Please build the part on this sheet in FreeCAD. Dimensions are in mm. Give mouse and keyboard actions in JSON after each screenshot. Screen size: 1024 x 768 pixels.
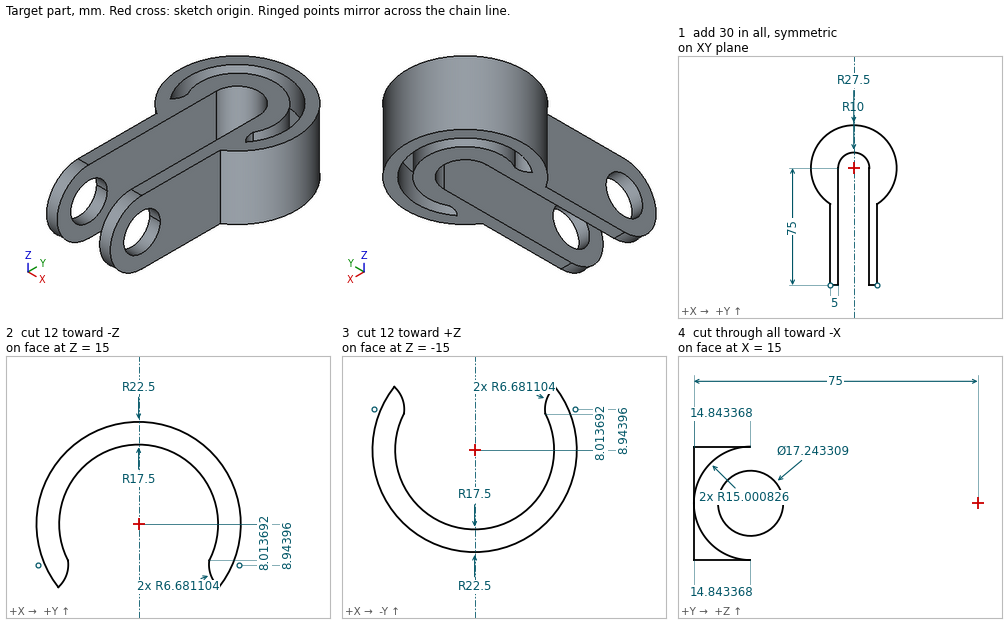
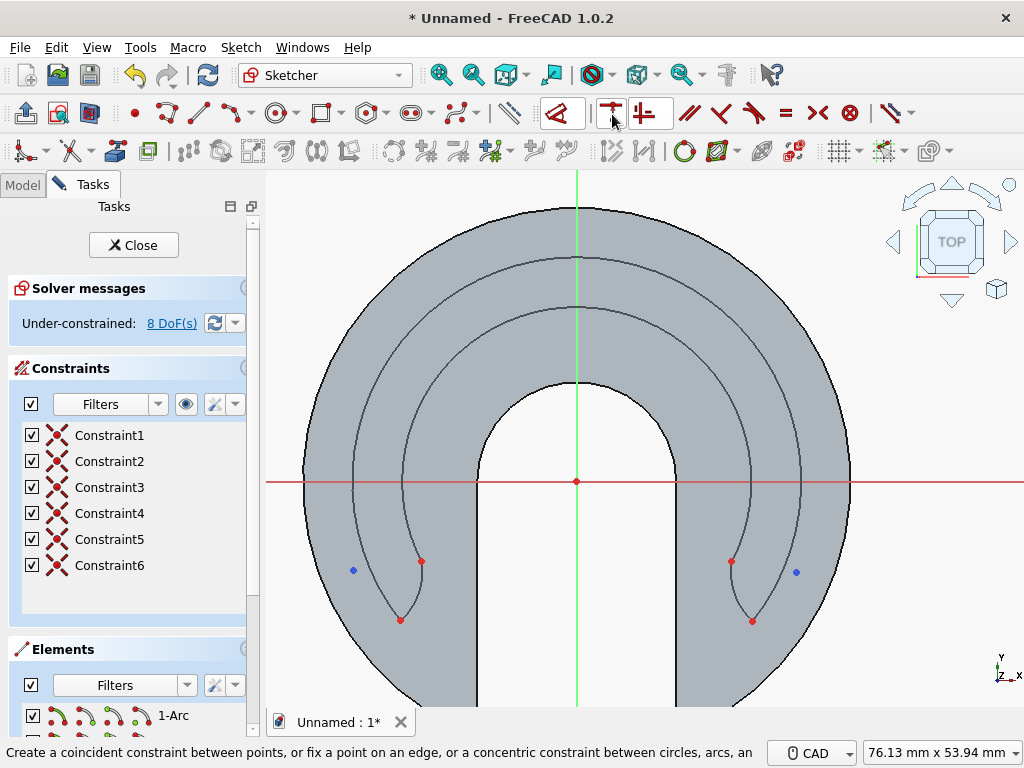
{"action": "left_click", "coordinate": [732, 582]}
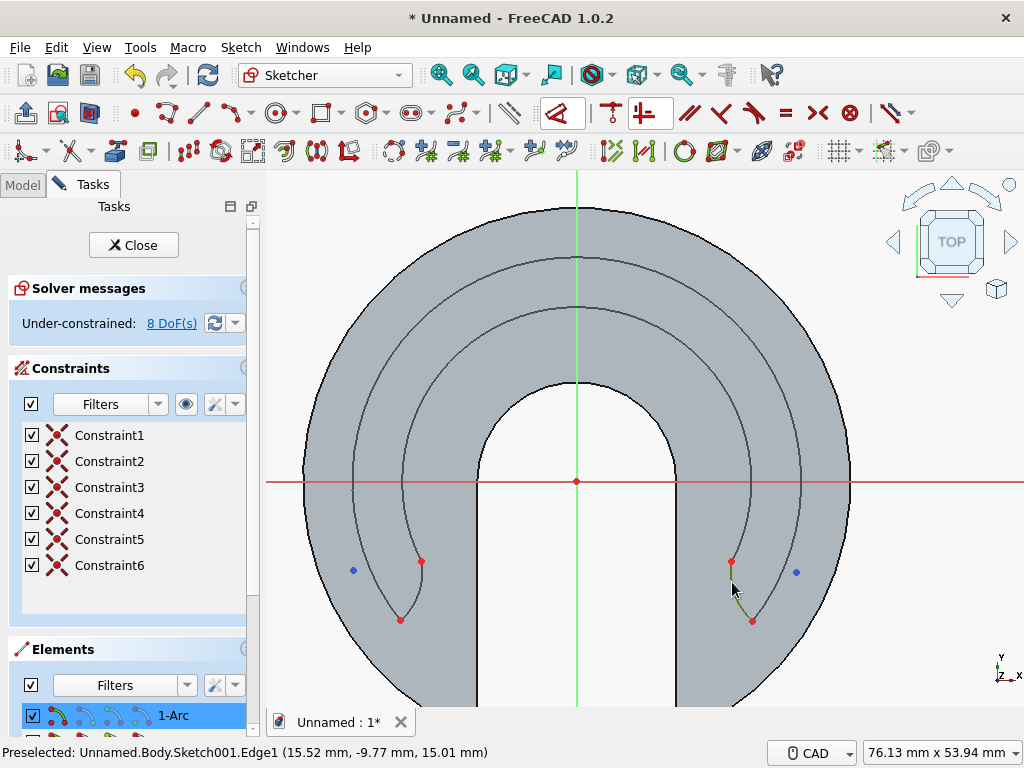
{"action": "left_click", "coordinate": [413, 606]}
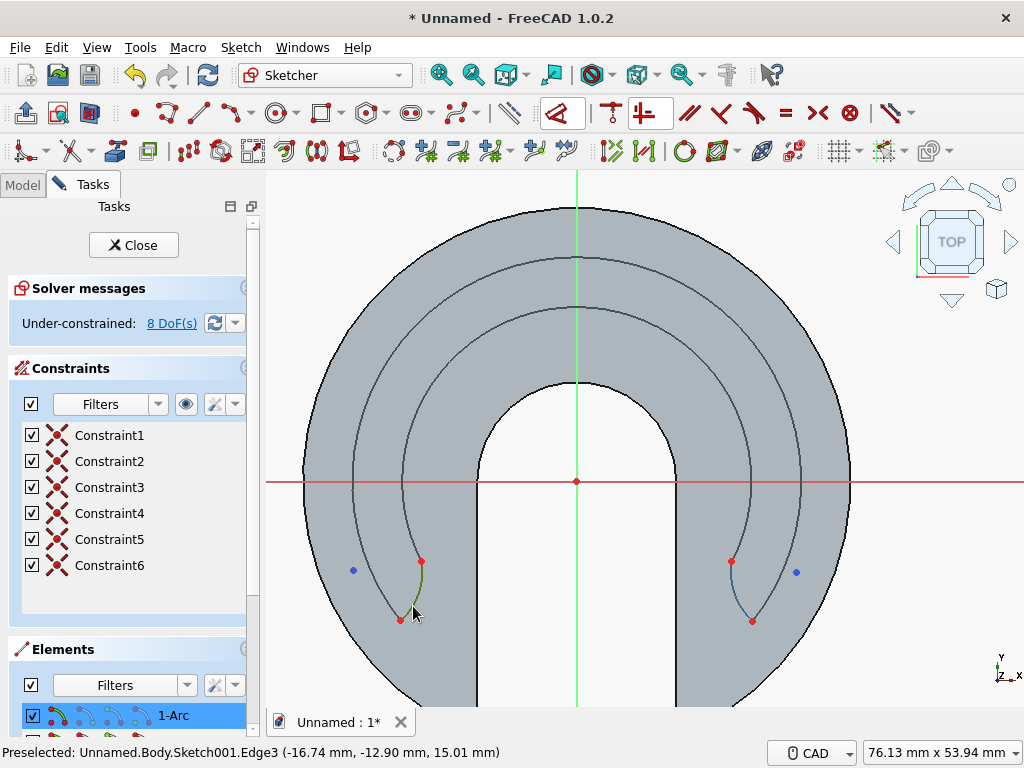
{"action": "left_click", "coordinate": [786, 114]}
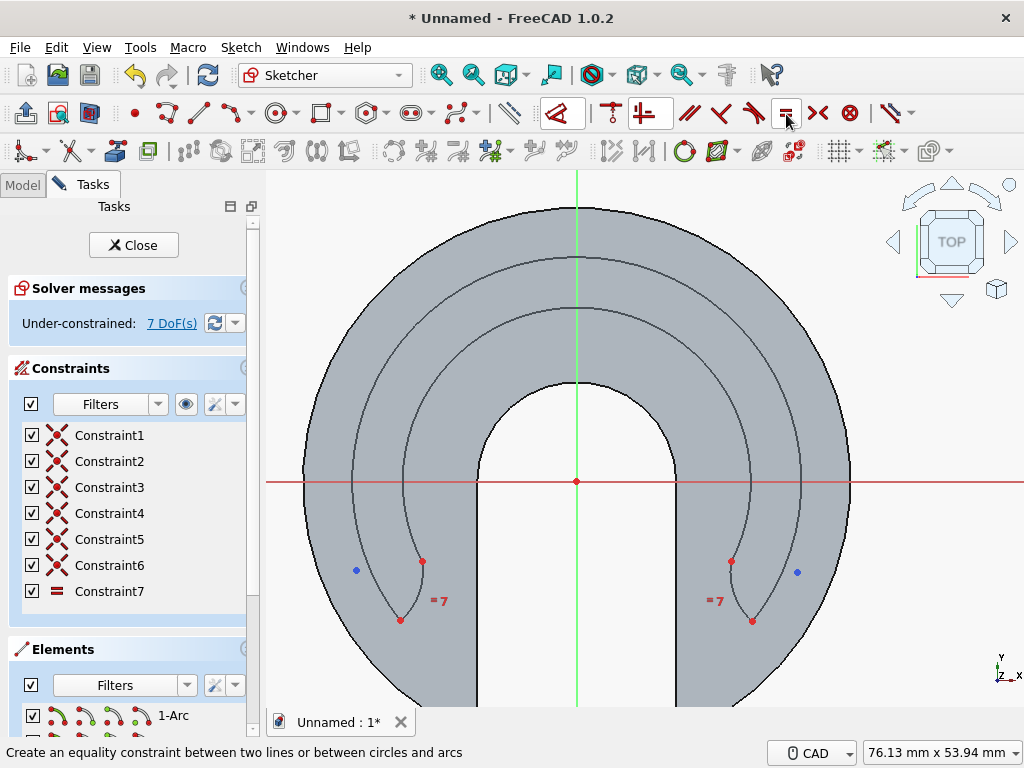
{"action": "left_click", "coordinate": [797, 572]}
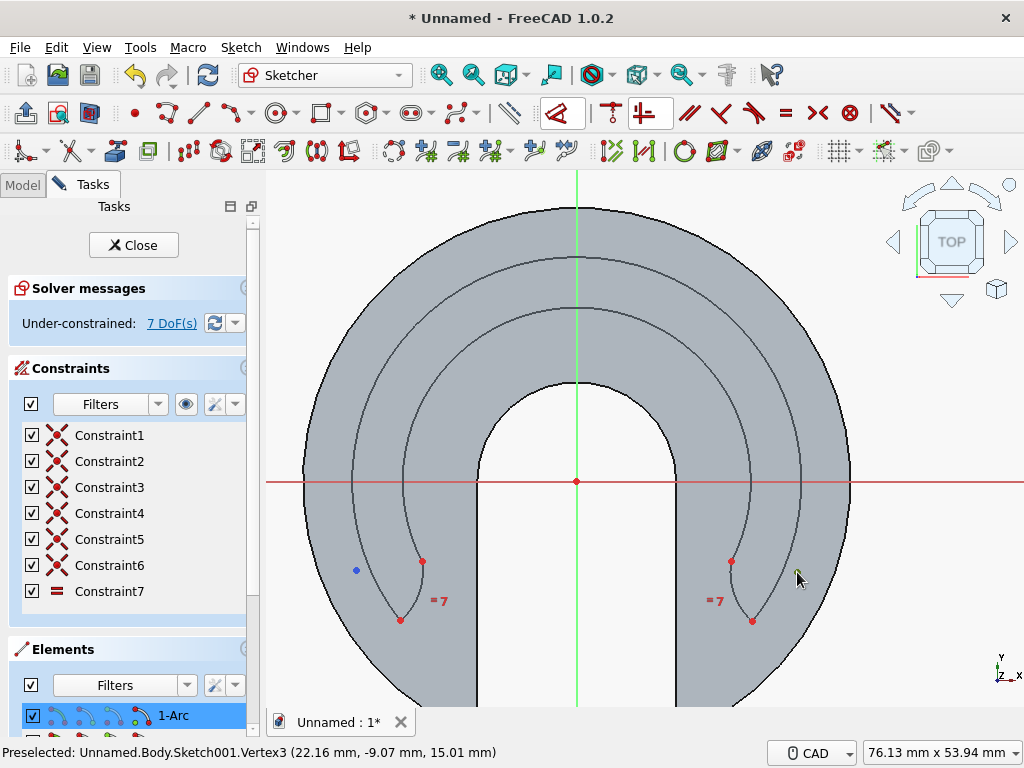
{"action": "left_click", "coordinate": [356, 571]}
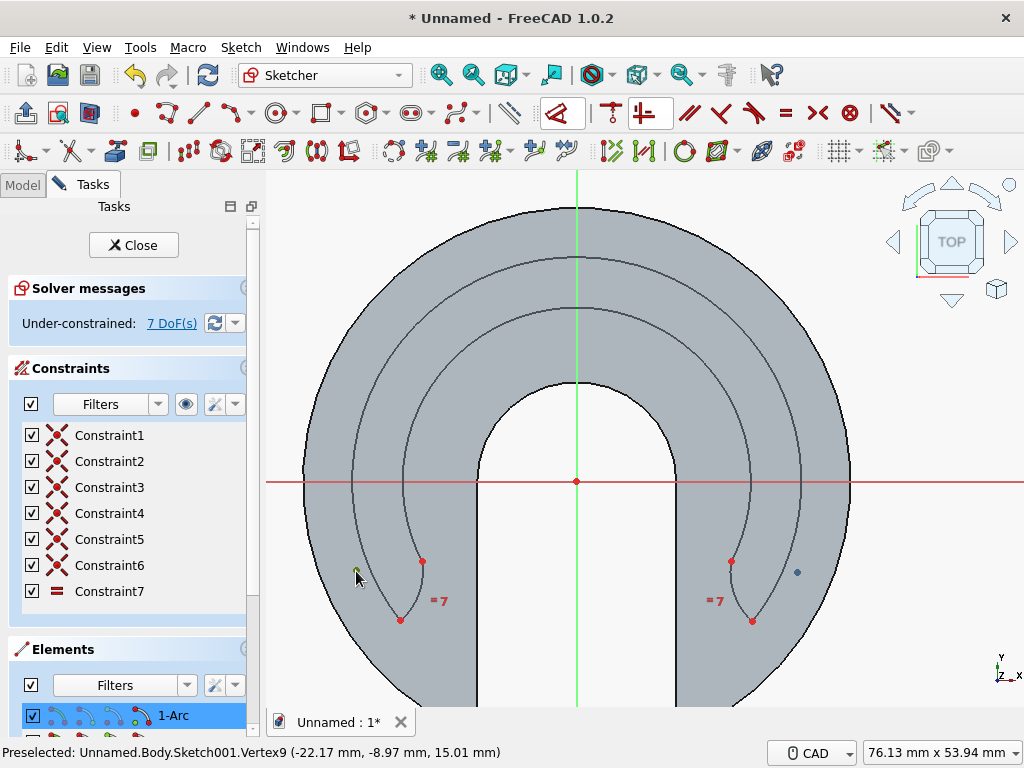
{"action": "left_click", "coordinate": [577, 645]}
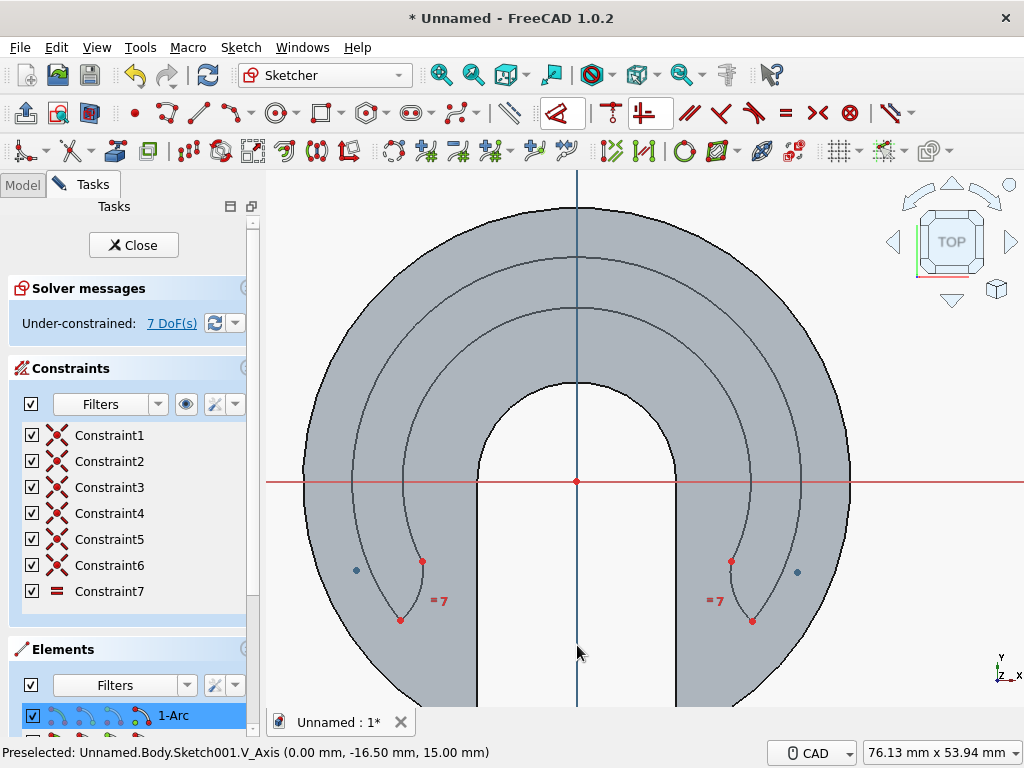
{"action": "key", "text": "s"}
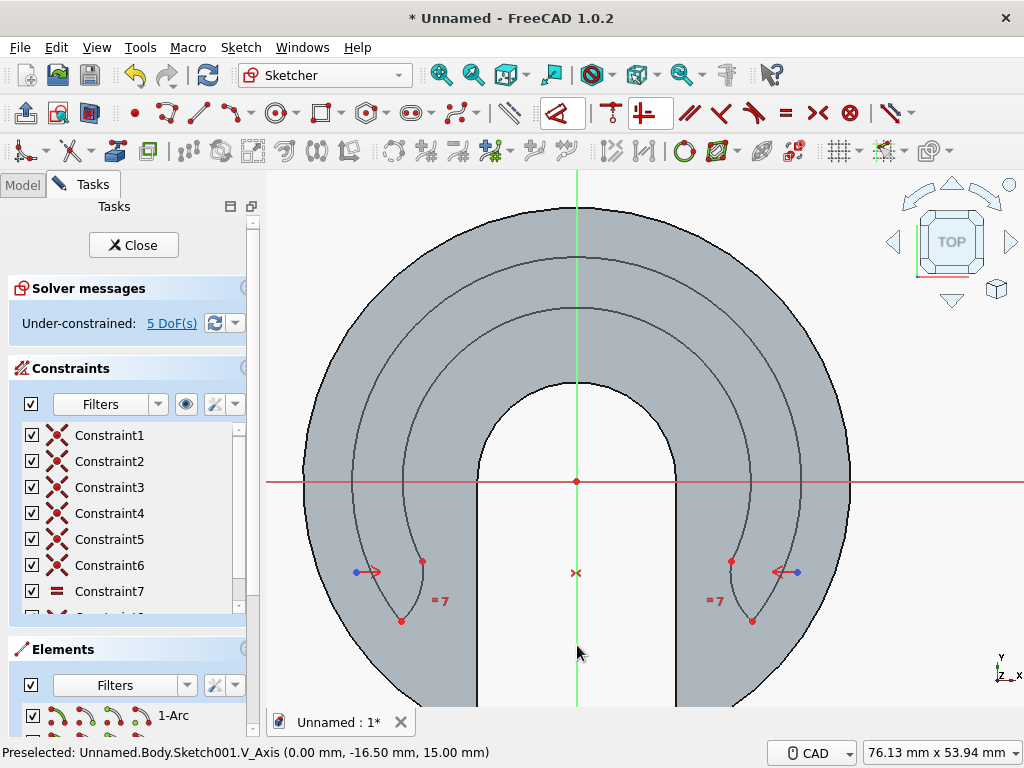
{"action": "left_click", "coordinate": [731, 582]}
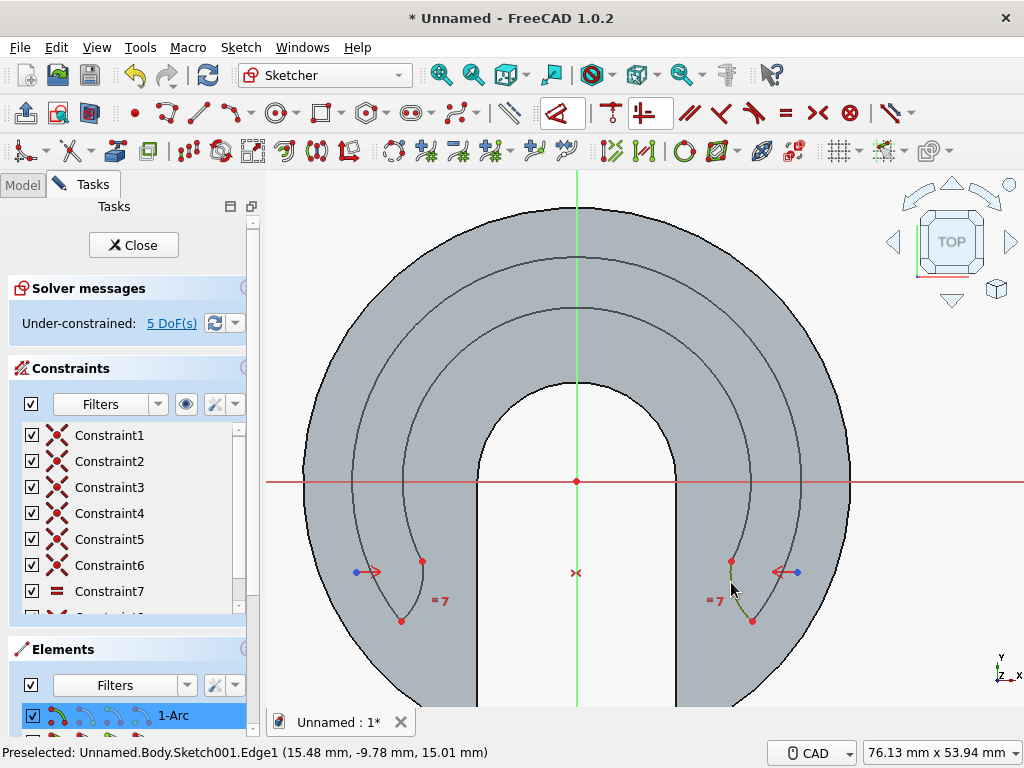
{"action": "left_click", "coordinate": [580, 114]}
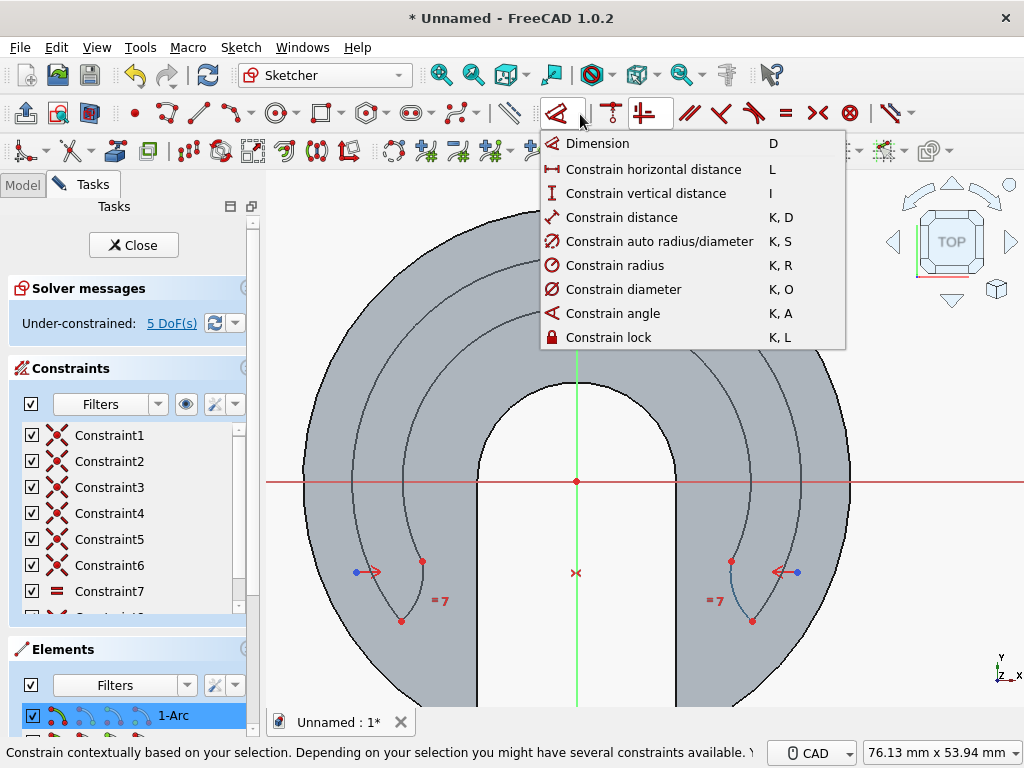
{"action": "left_click", "coordinate": [693, 265]}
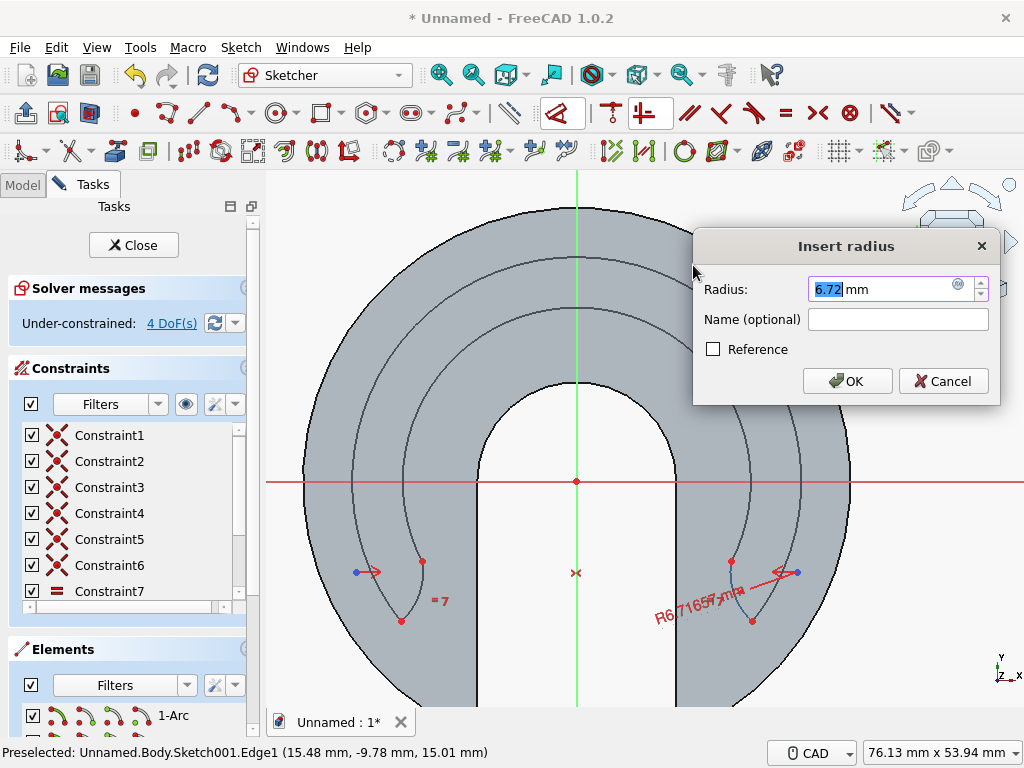
{"action": "type", "text": "6.681104"}
{"action": "key", "text": "Return"}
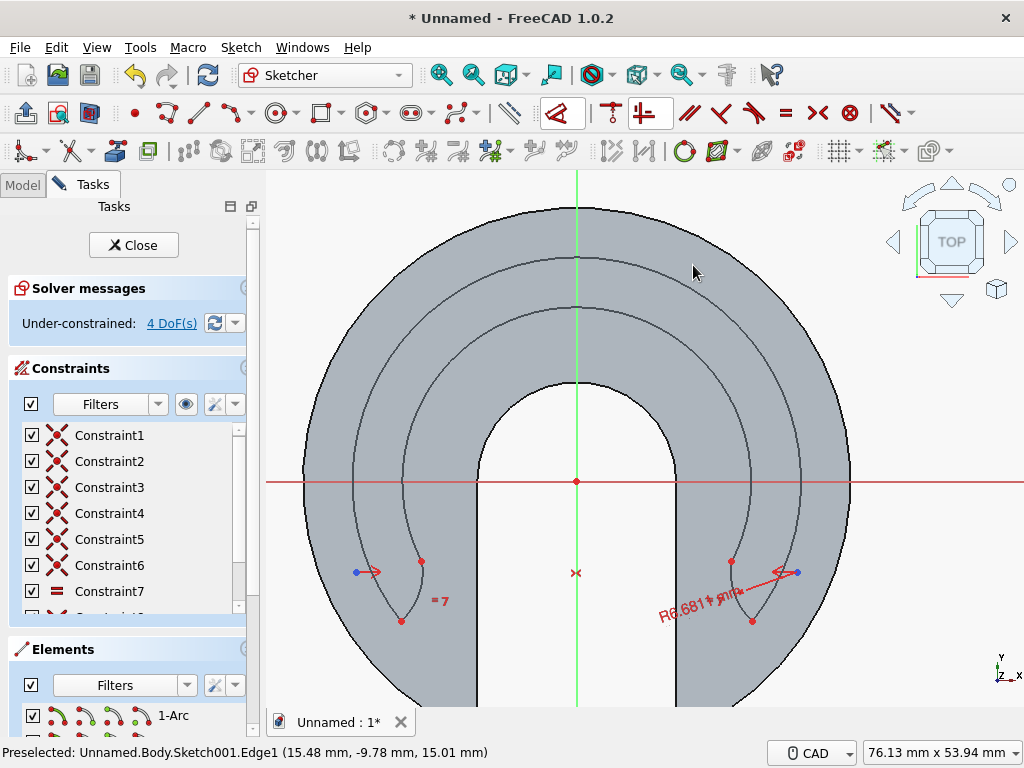
{"action": "left_click", "coordinate": [752, 342]}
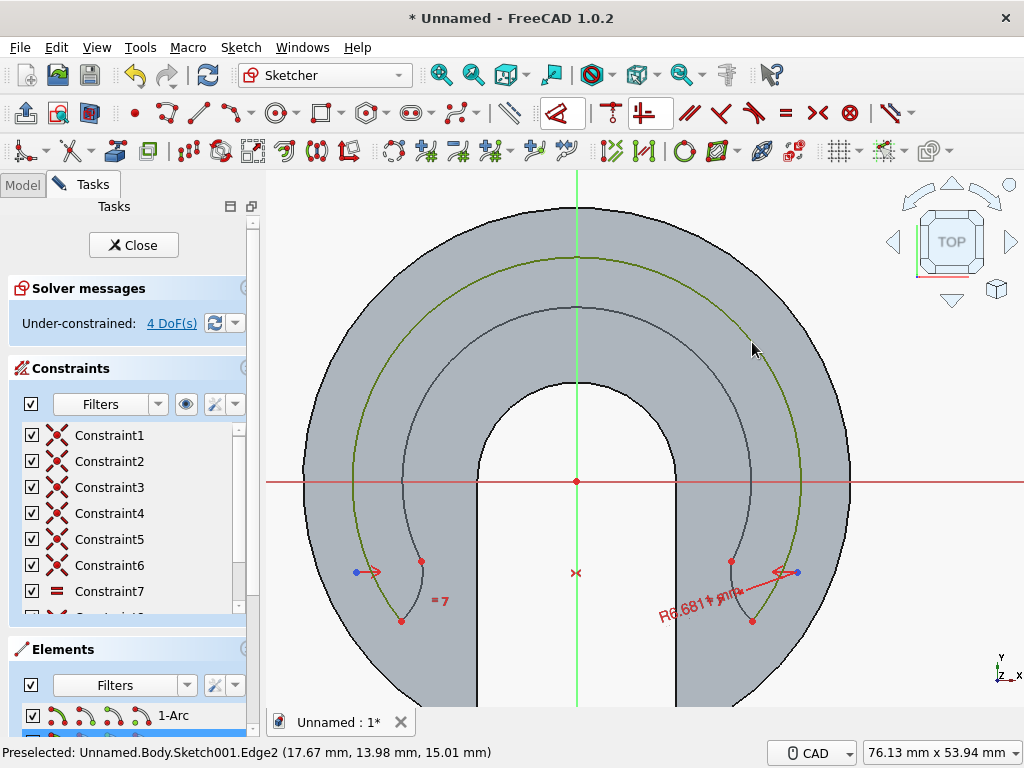
{"action": "key", "text": "k r"}